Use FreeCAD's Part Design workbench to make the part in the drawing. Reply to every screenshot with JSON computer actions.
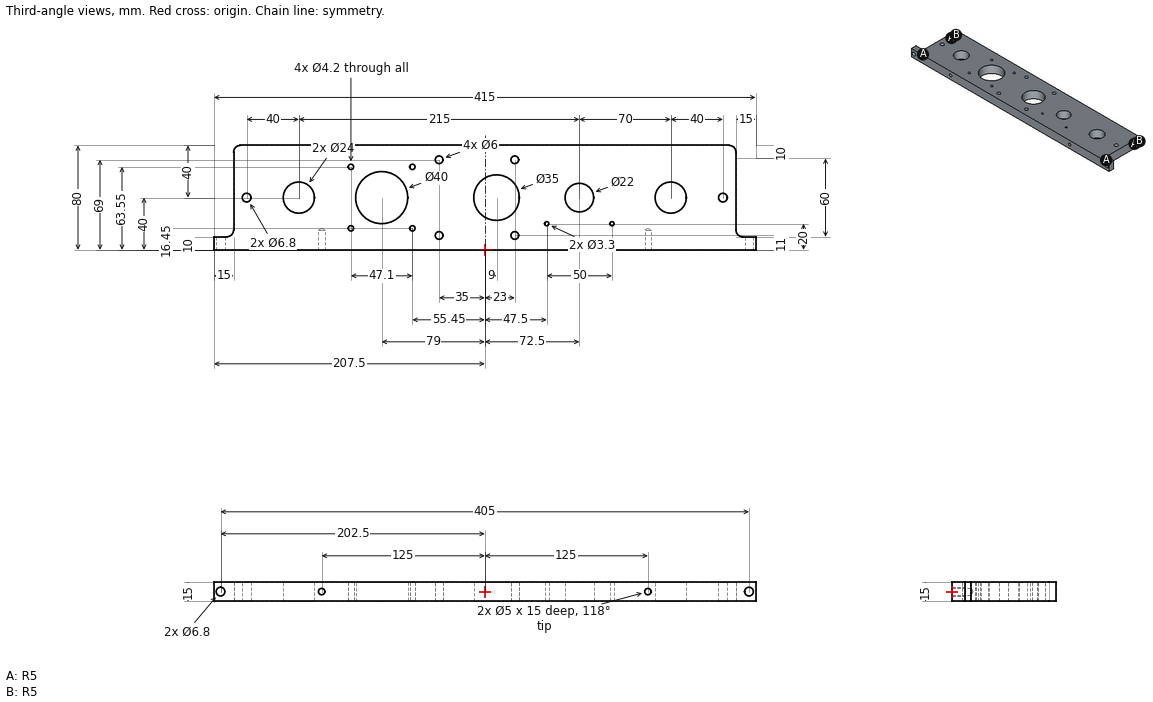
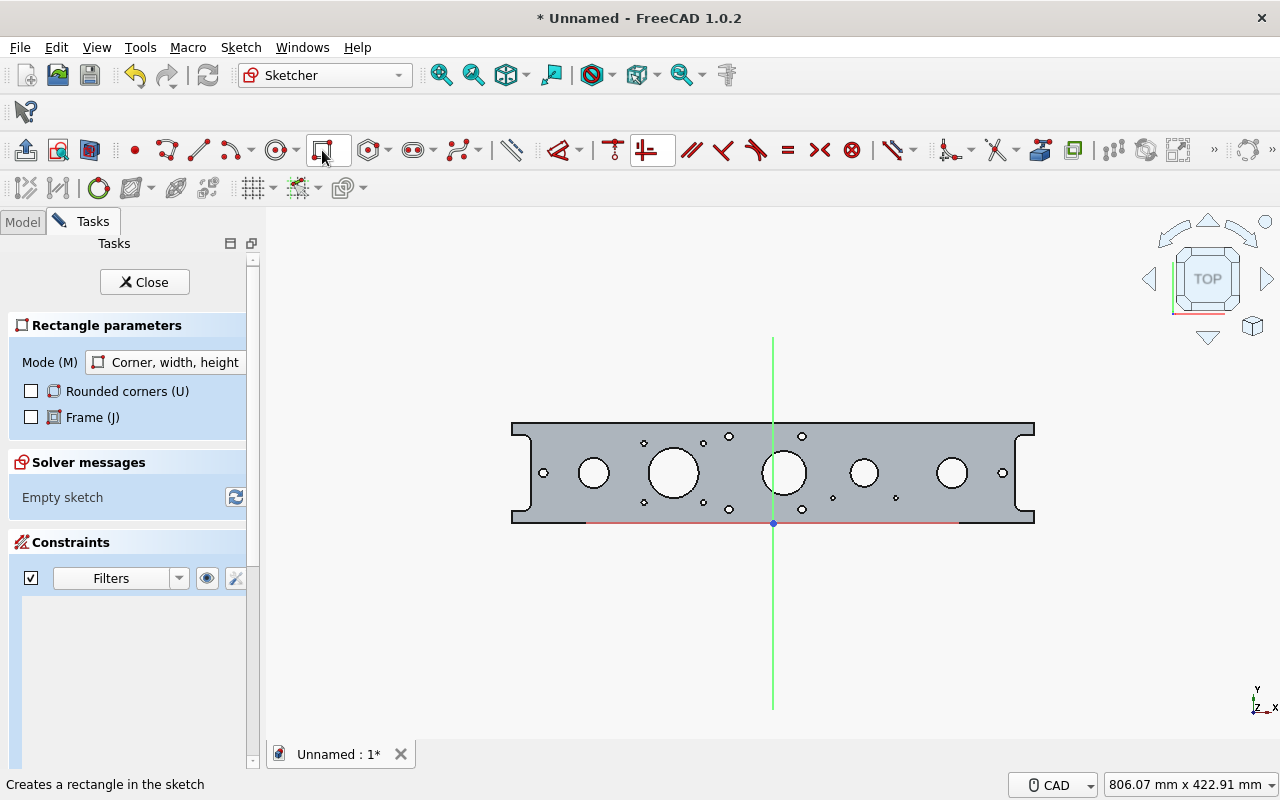
{"action": "left_click", "coordinate": [512, 423]}
{"action": "left_click", "coordinate": [531, 473]}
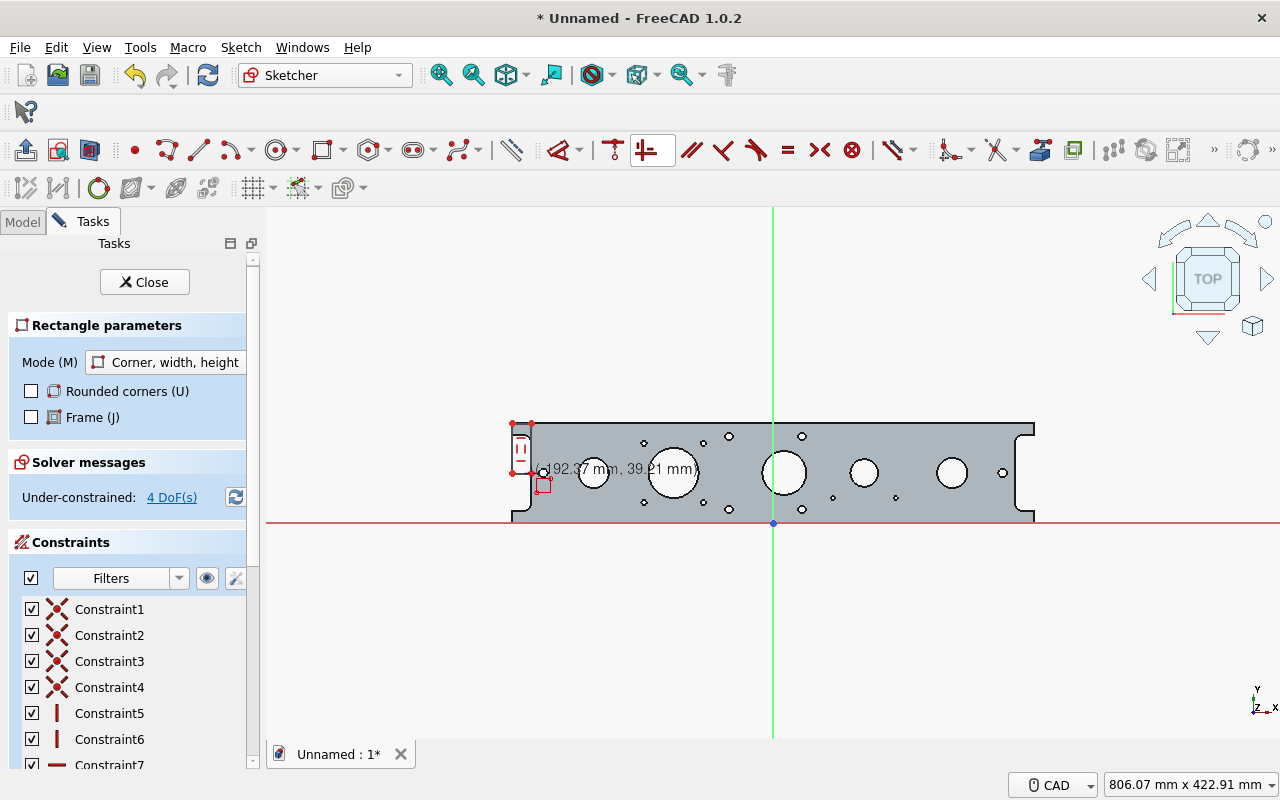
{"action": "left_click", "coordinate": [1015, 423]}
{"action": "left_click", "coordinate": [1034, 473]}
{"action": "key", "text": "Escape"}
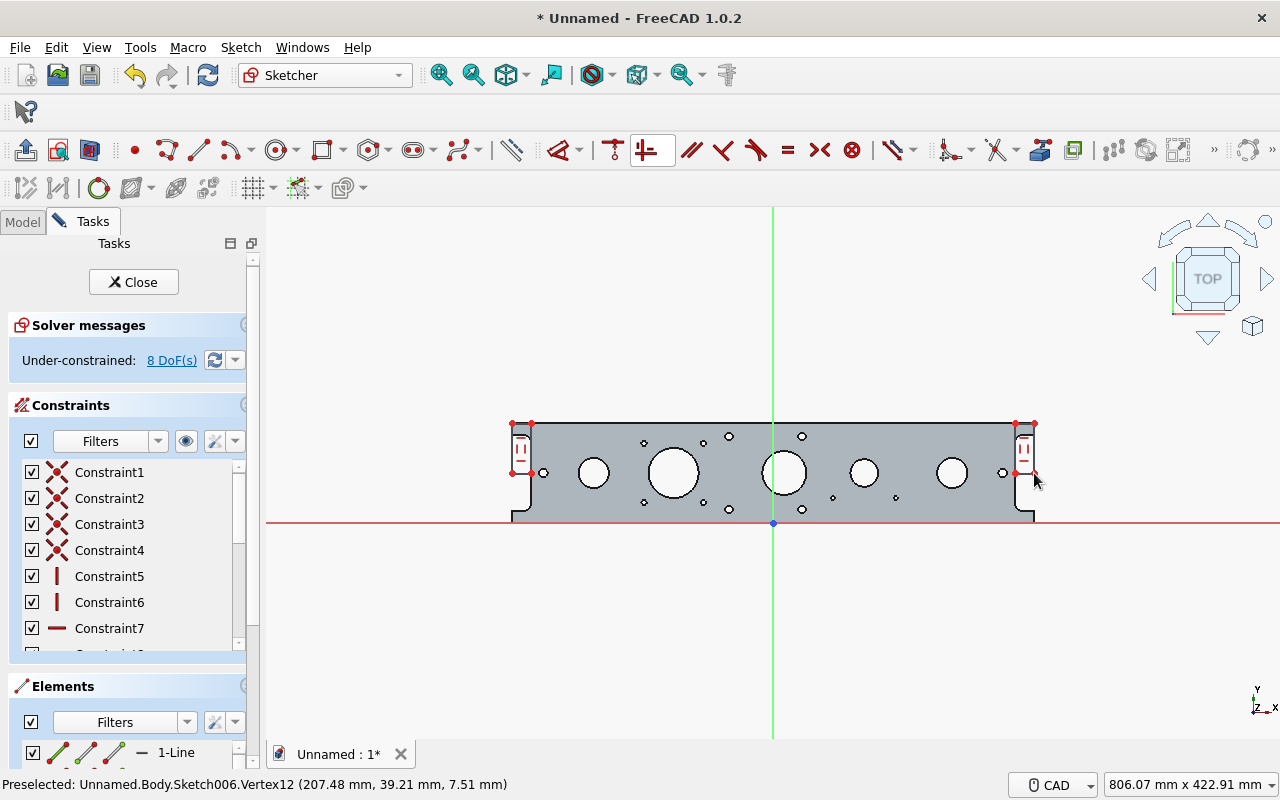
{"action": "left_click", "coordinate": [531, 424]}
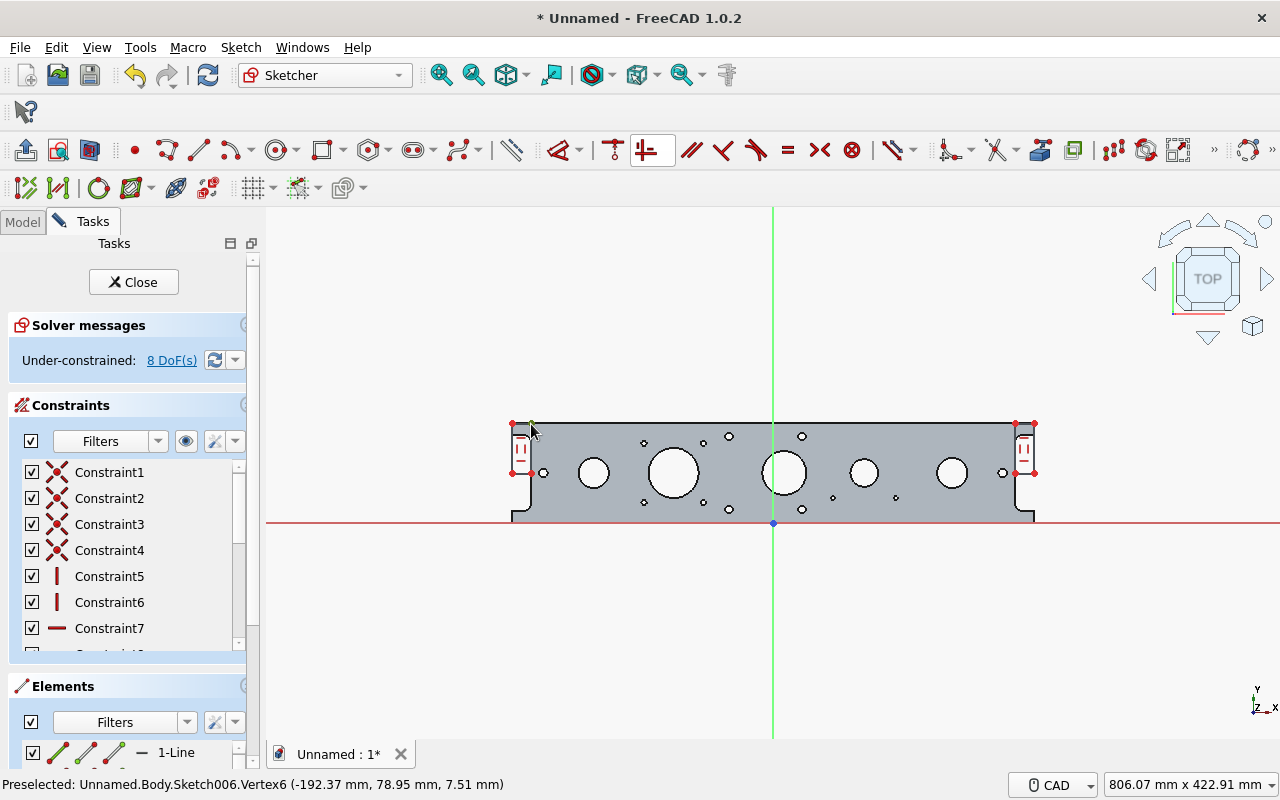
{"action": "left_click", "coordinate": [1015, 424]}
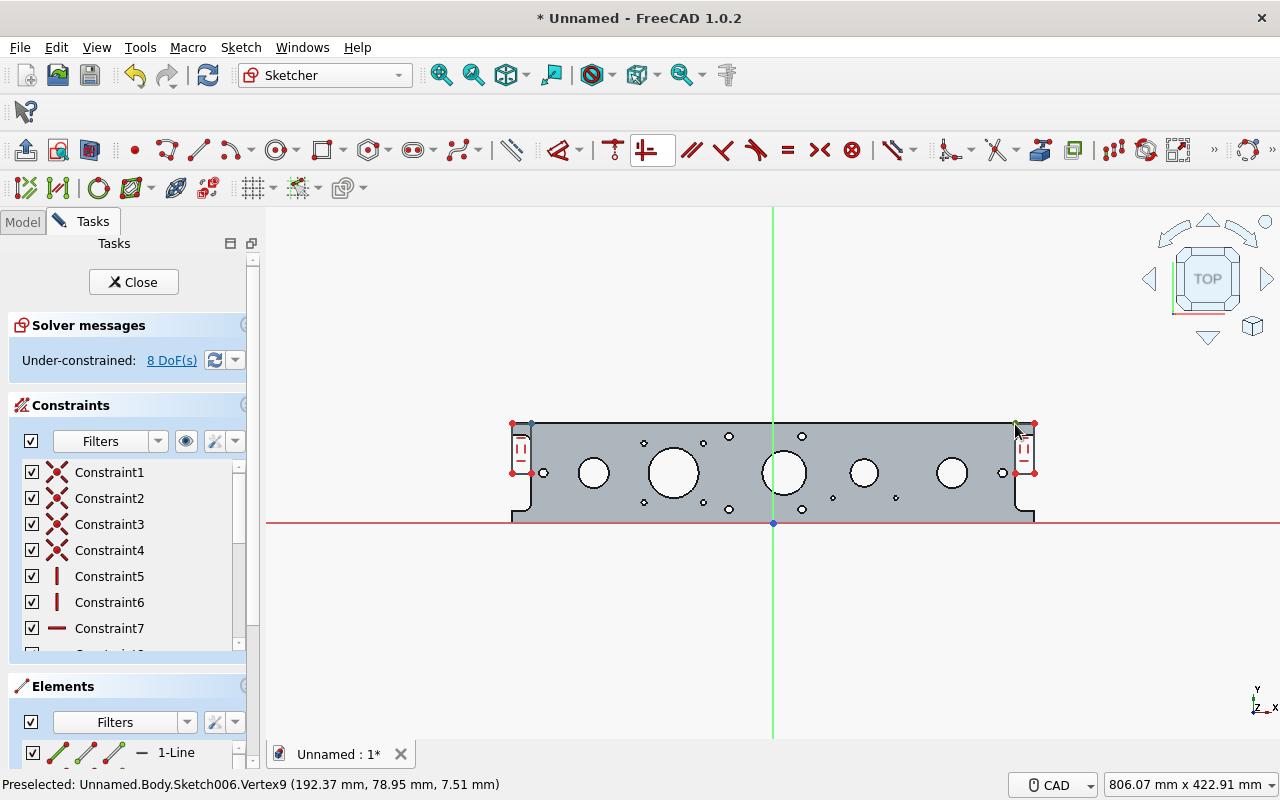
{"action": "left_click", "coordinate": [773, 677]}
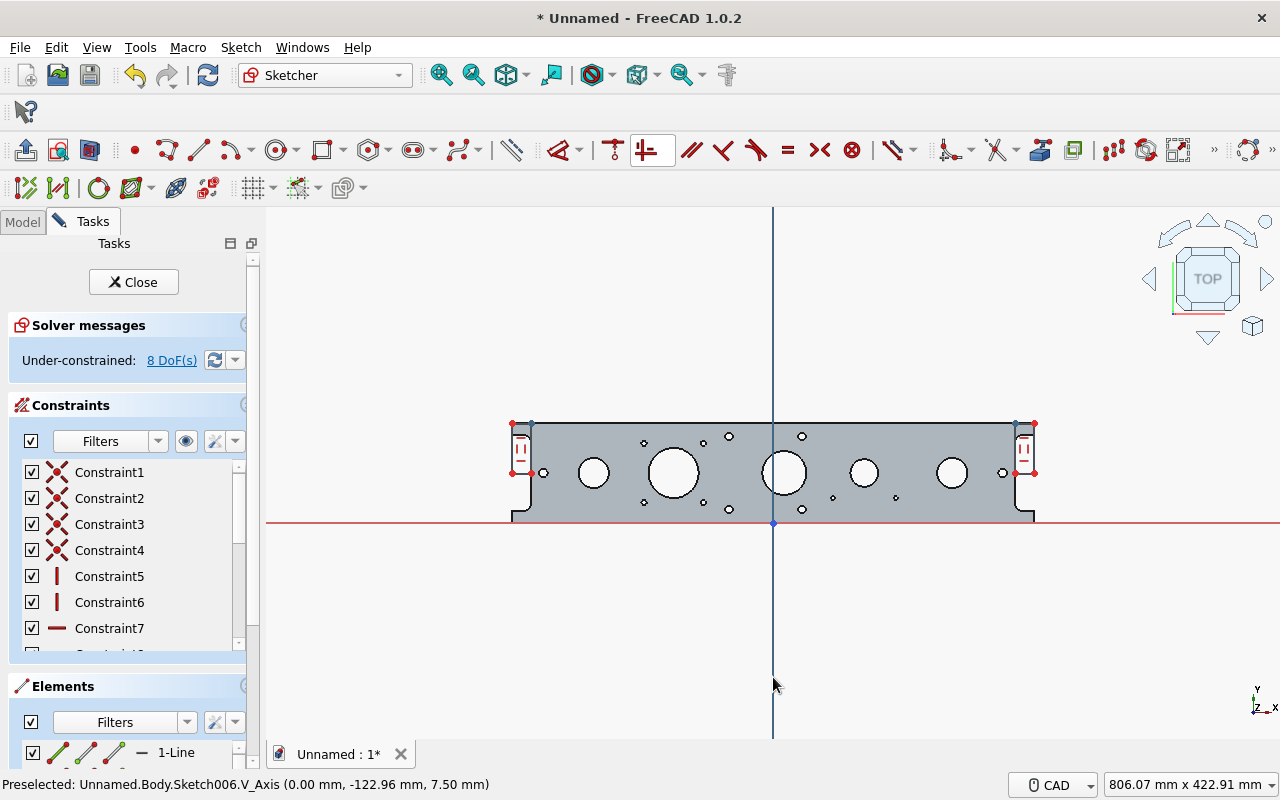
{"action": "left_click", "coordinate": [820, 150]}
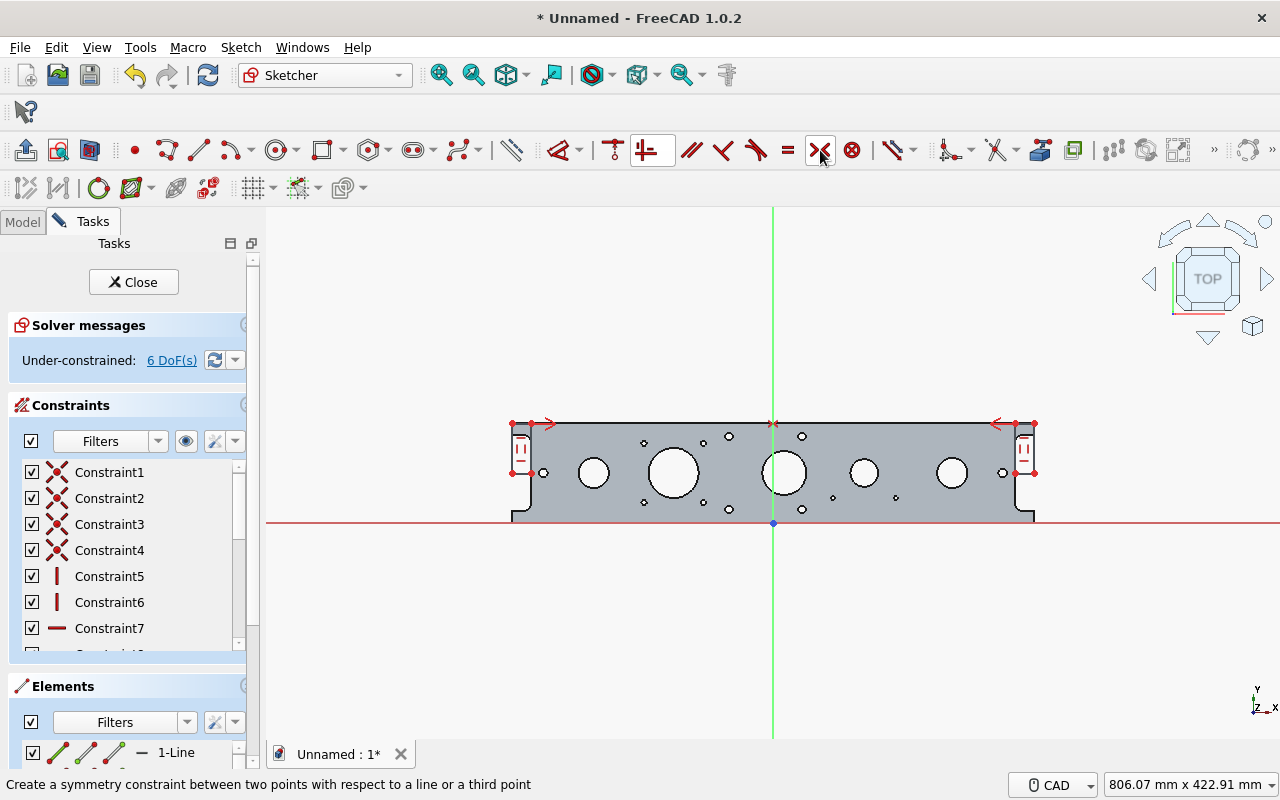
{"action": "left_click", "coordinate": [512, 474]}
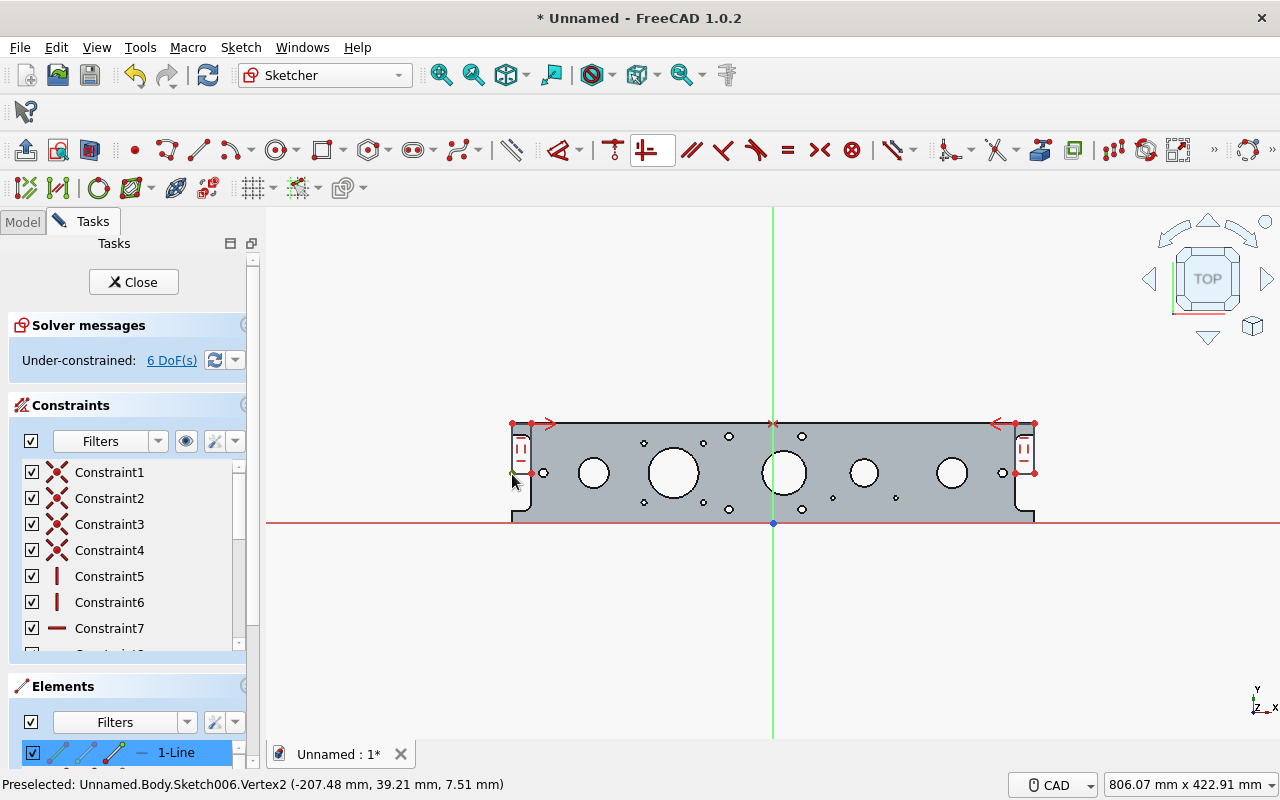
{"action": "left_click", "coordinate": [1034, 474]}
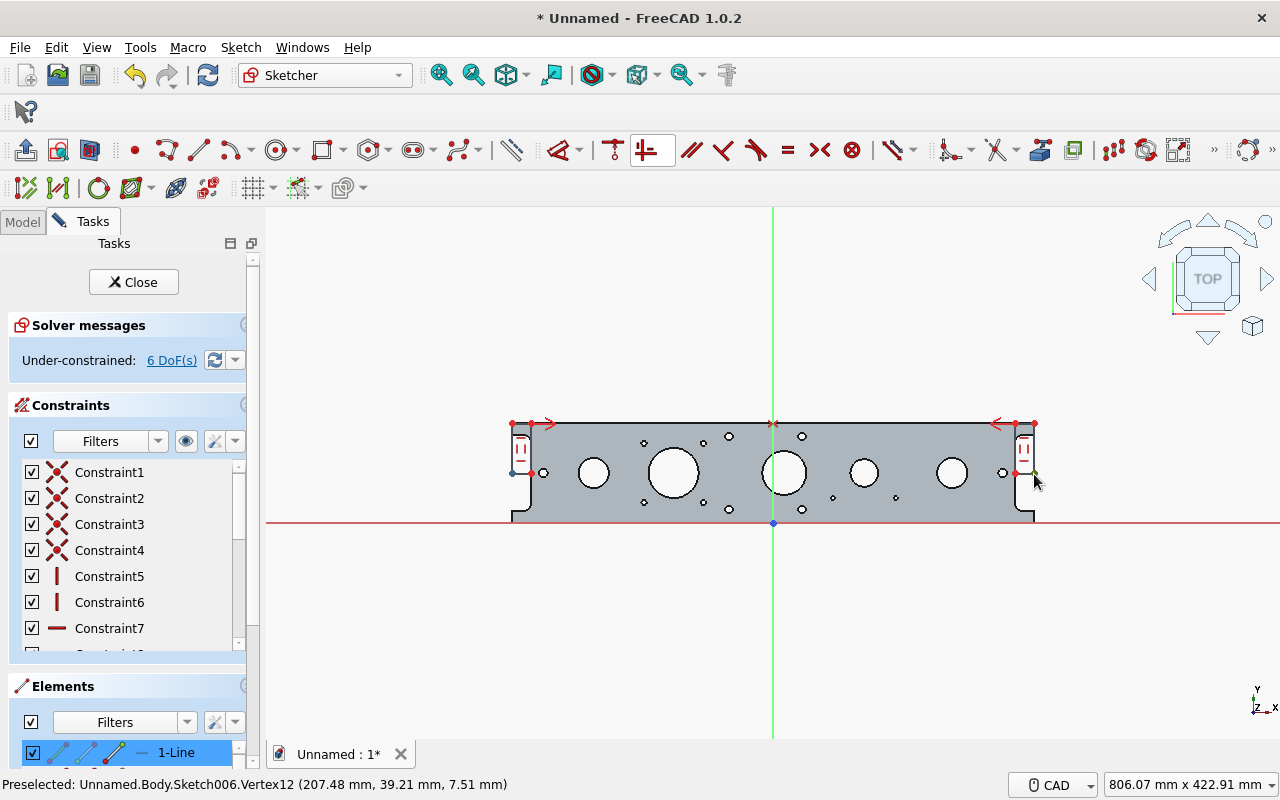
{"action": "left_click", "coordinate": [773, 677]}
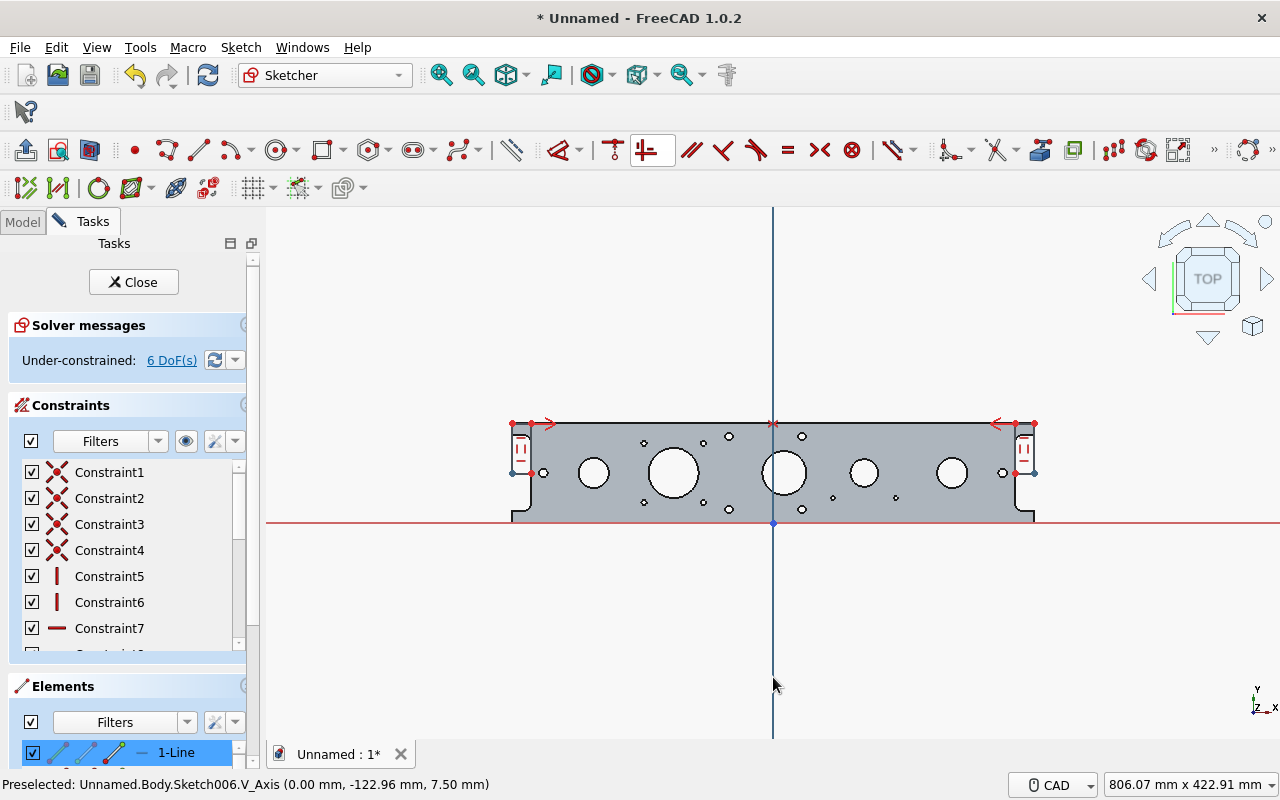
{"action": "left_click", "coordinate": [820, 150]}